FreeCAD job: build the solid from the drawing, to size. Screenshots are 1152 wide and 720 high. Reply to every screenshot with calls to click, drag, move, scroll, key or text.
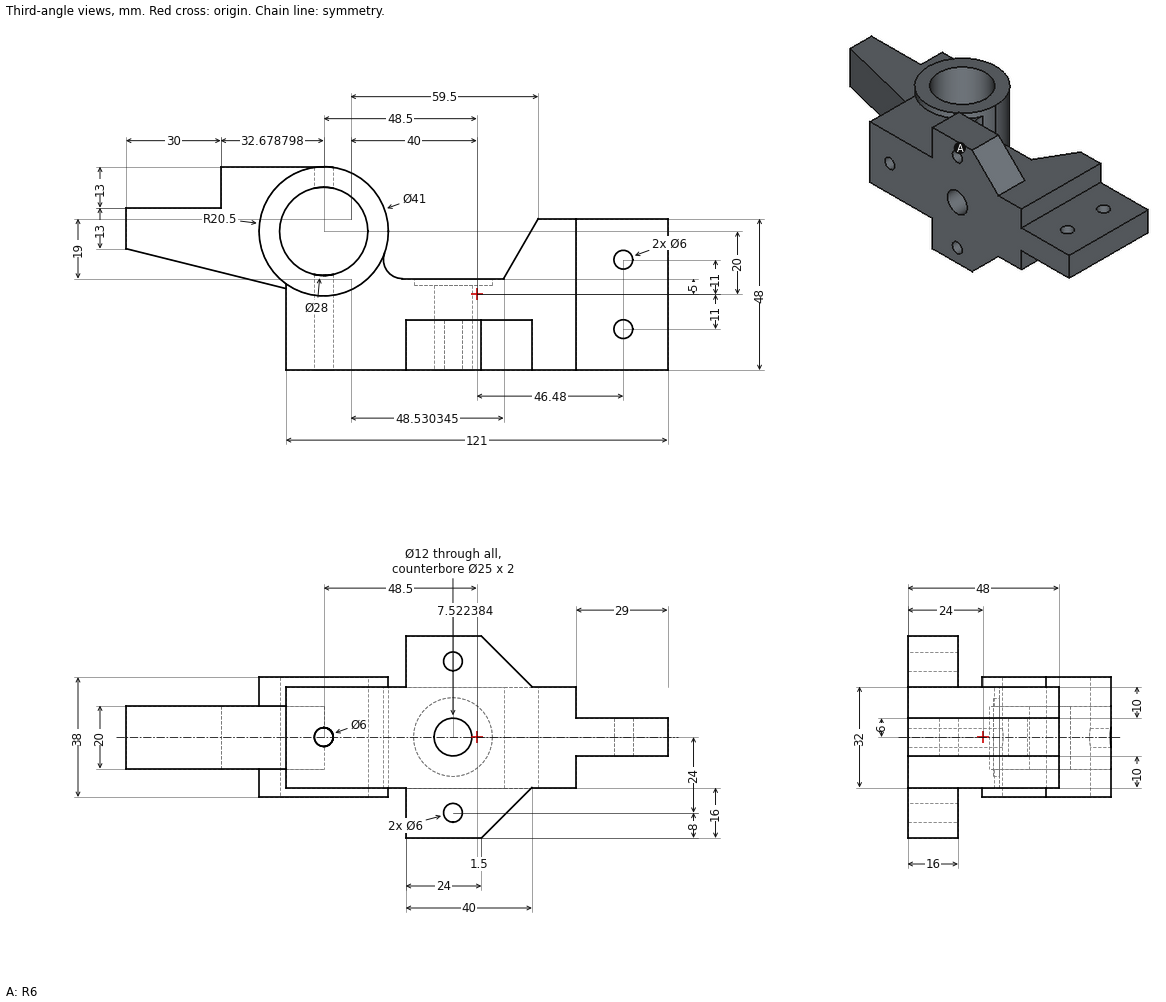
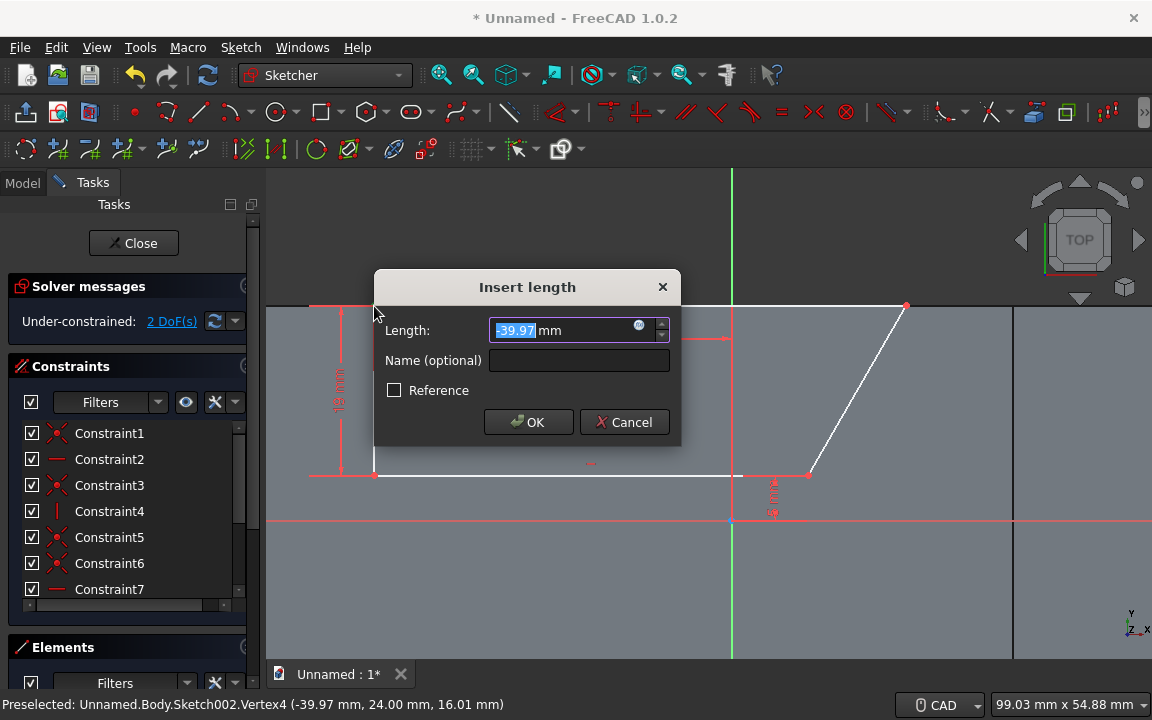
text(-40)
key(Return)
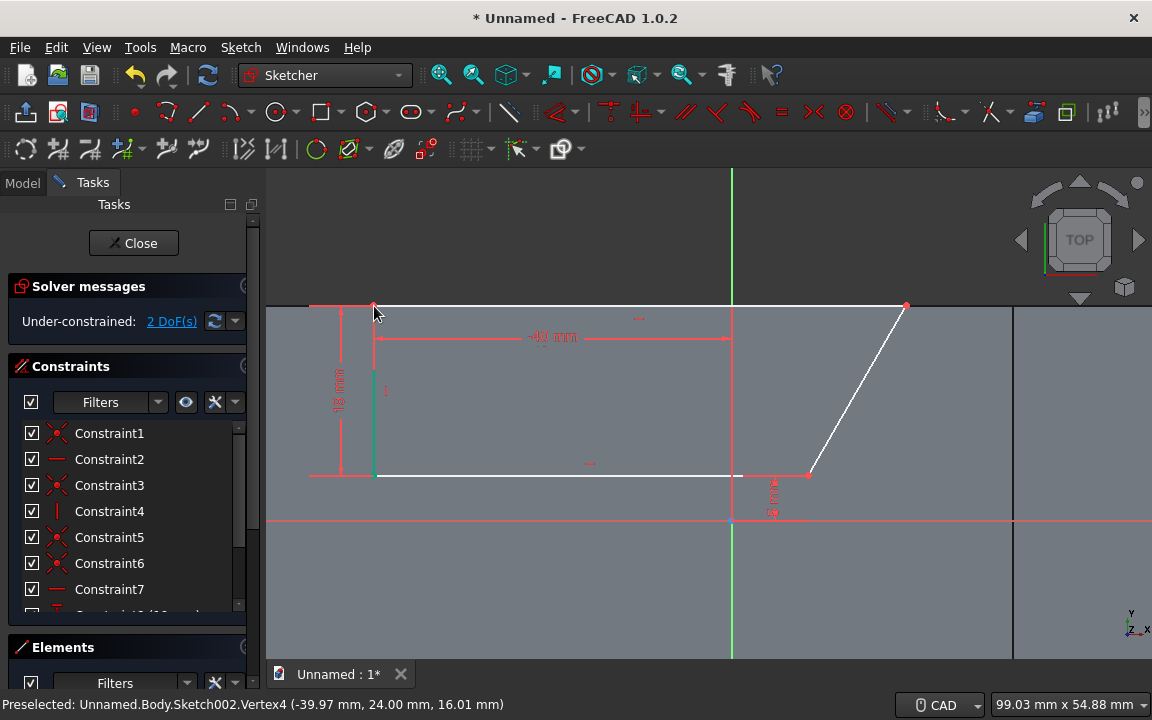
click(746, 306)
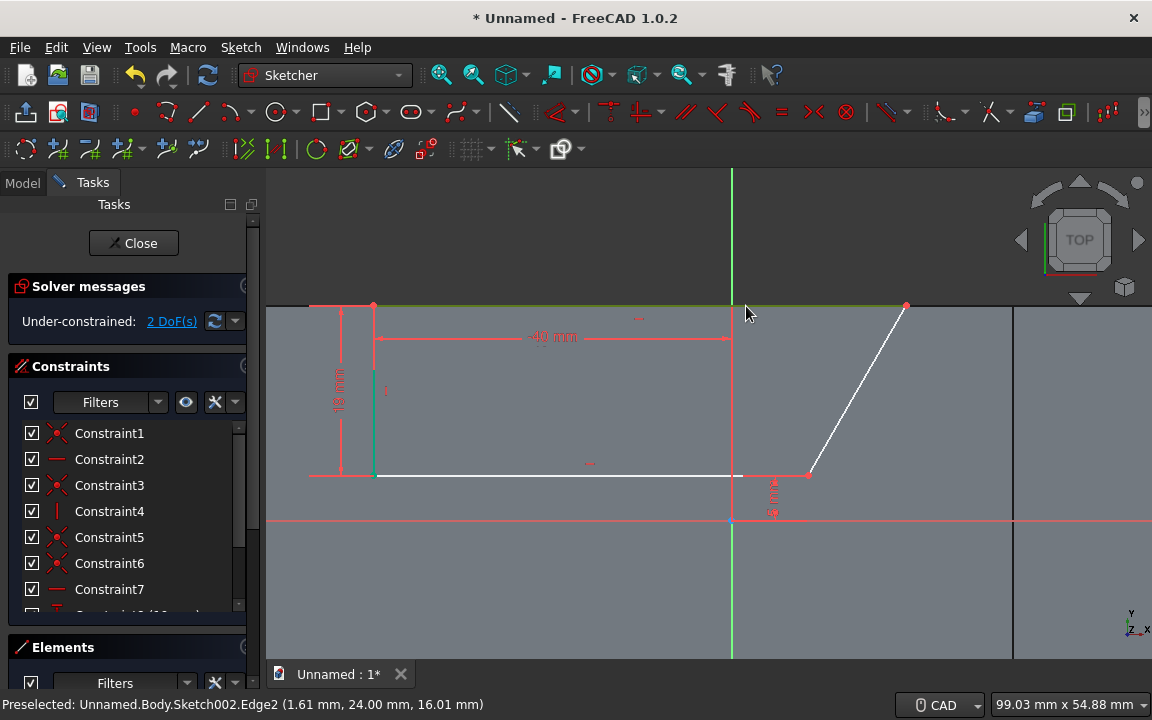
click(578, 112)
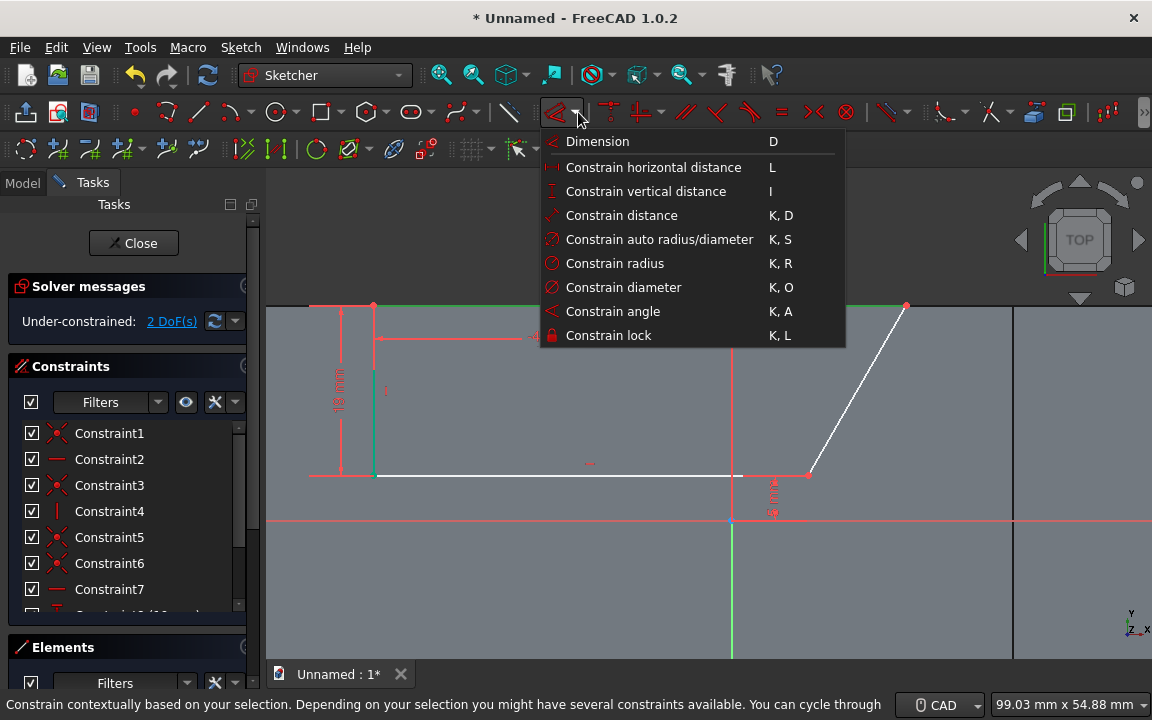
click(693, 167)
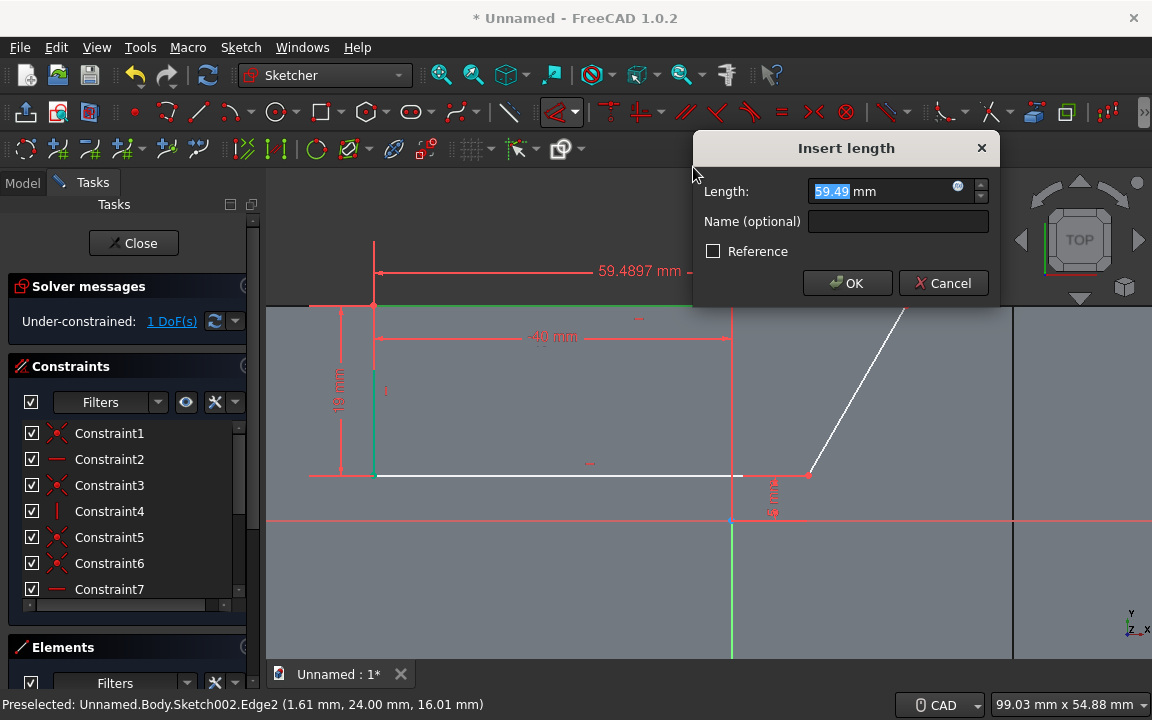
text(59.5)
key(Return)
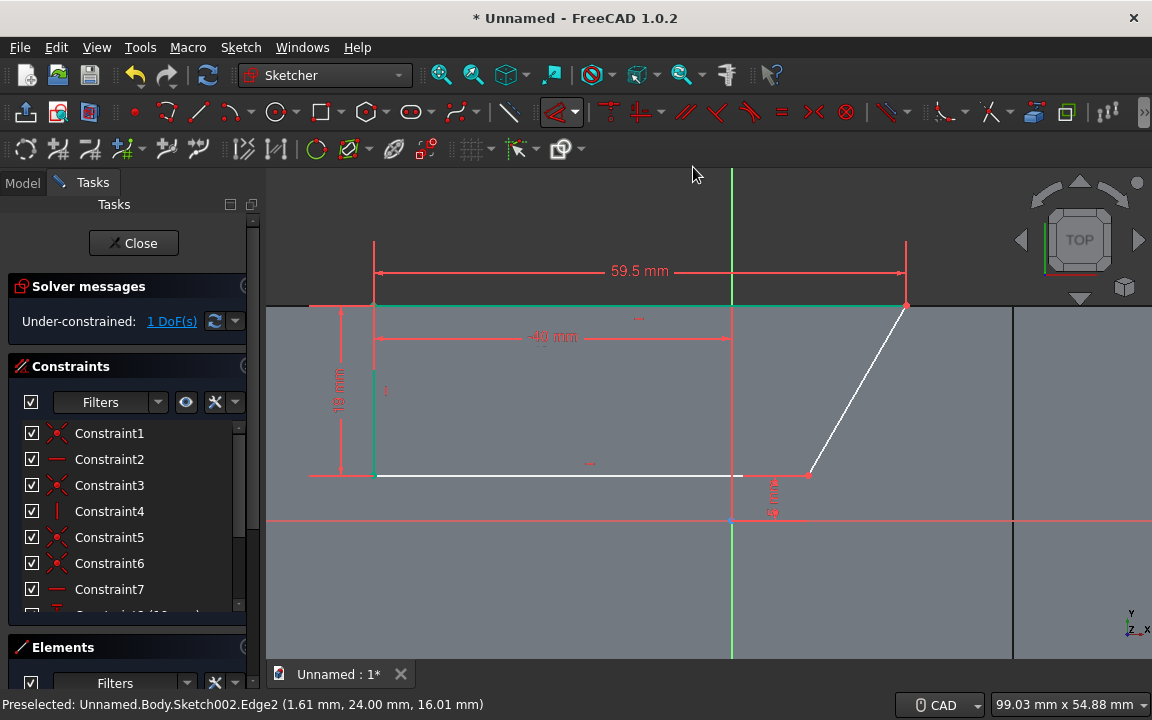
click(504, 476)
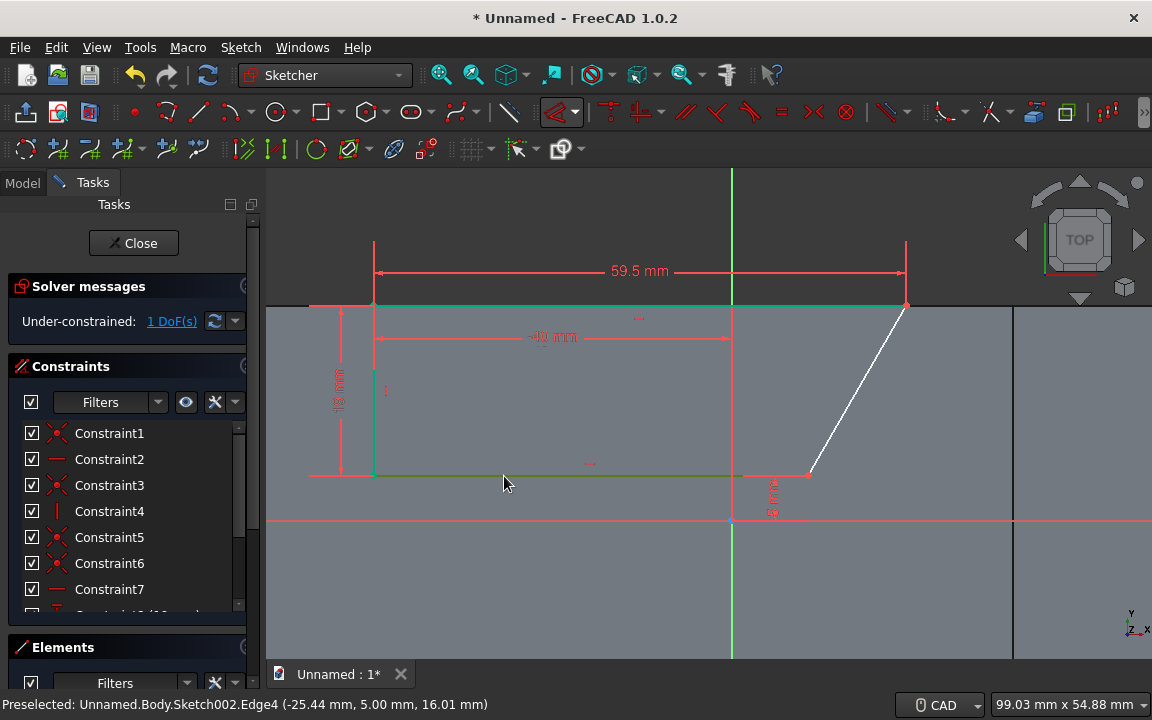
key(l)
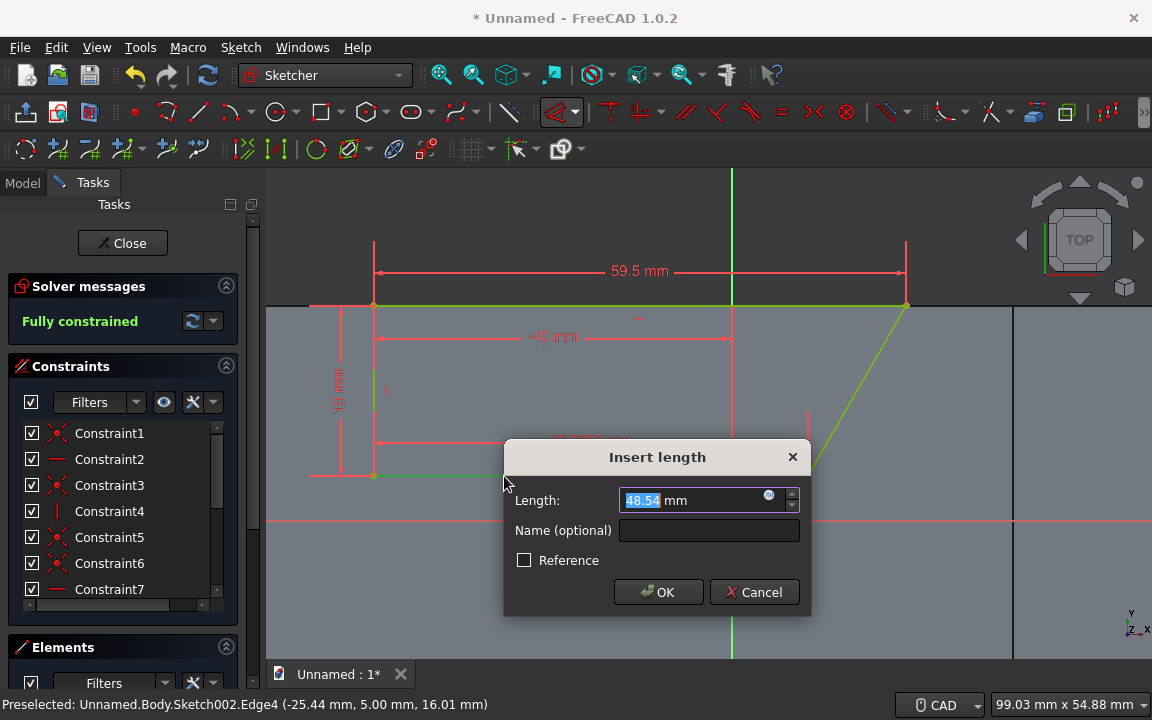
text(48.530345)
key(Return)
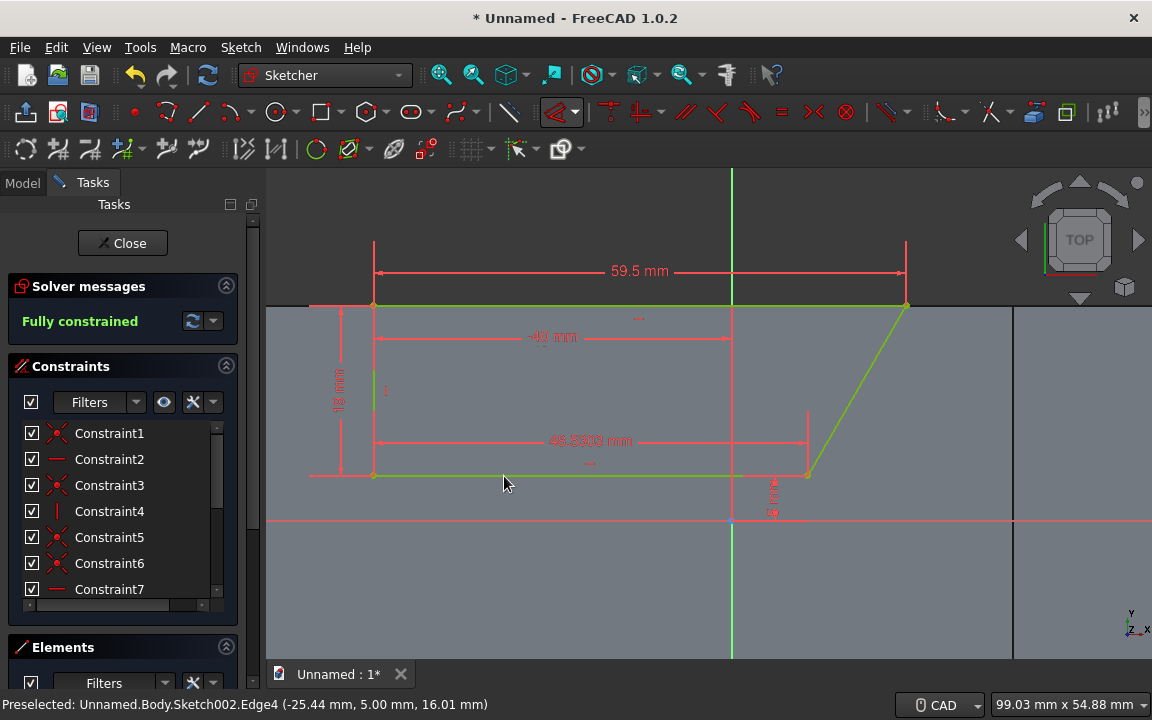
click(123, 243)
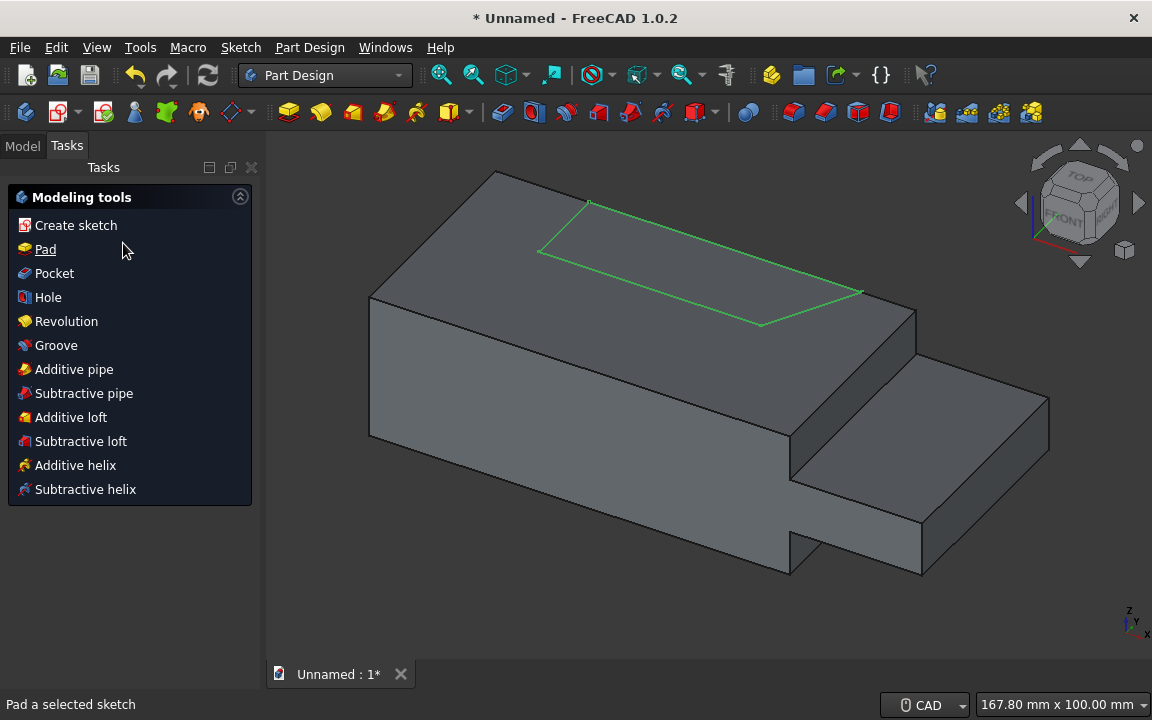
click(504, 112)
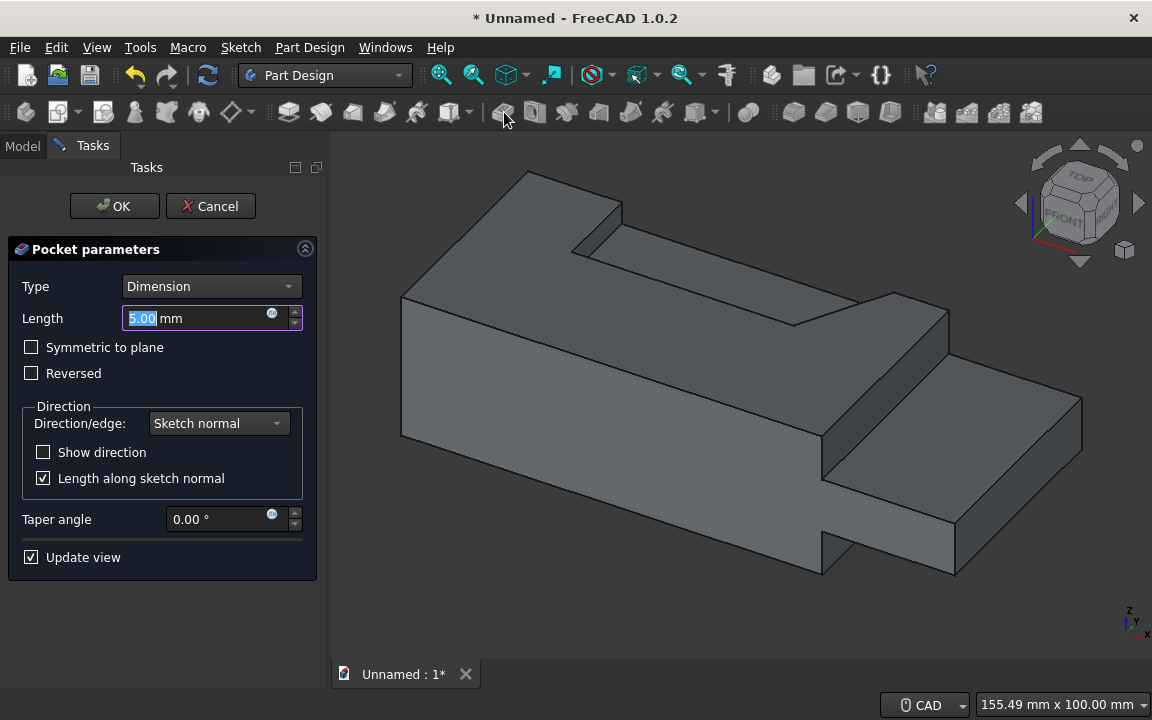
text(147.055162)
key(Tab)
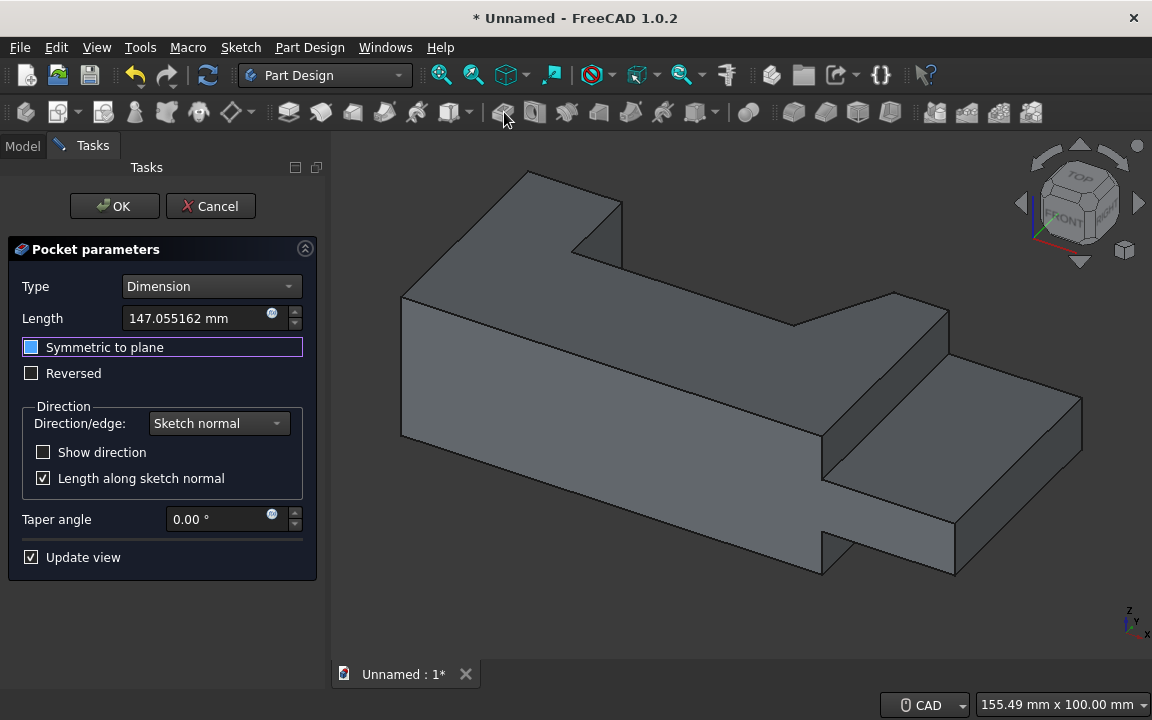
click(30, 347)